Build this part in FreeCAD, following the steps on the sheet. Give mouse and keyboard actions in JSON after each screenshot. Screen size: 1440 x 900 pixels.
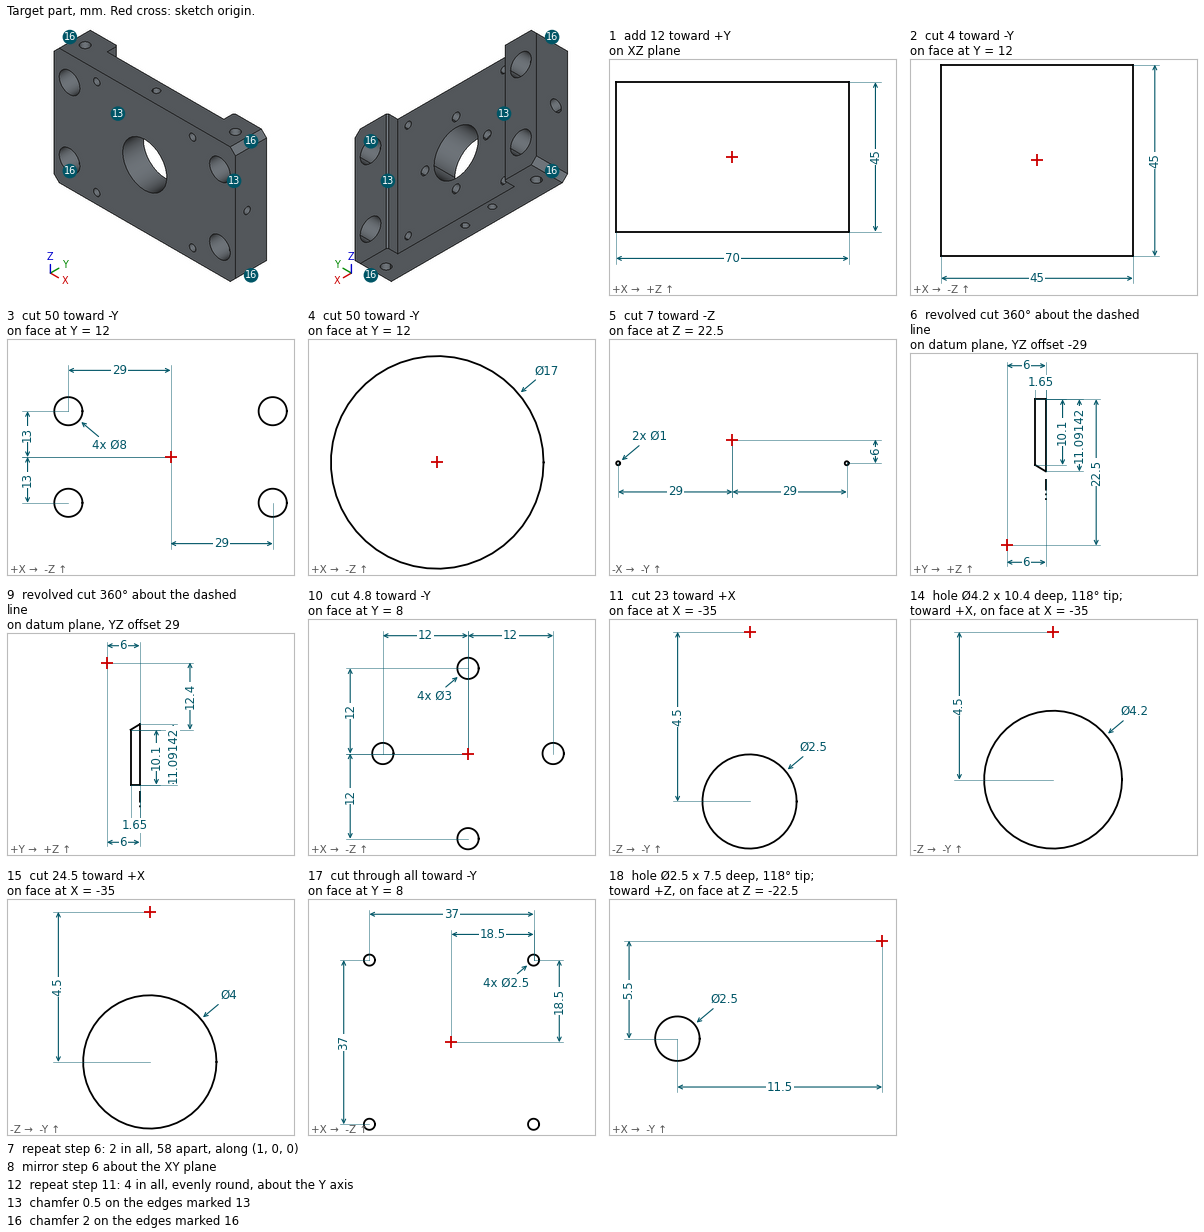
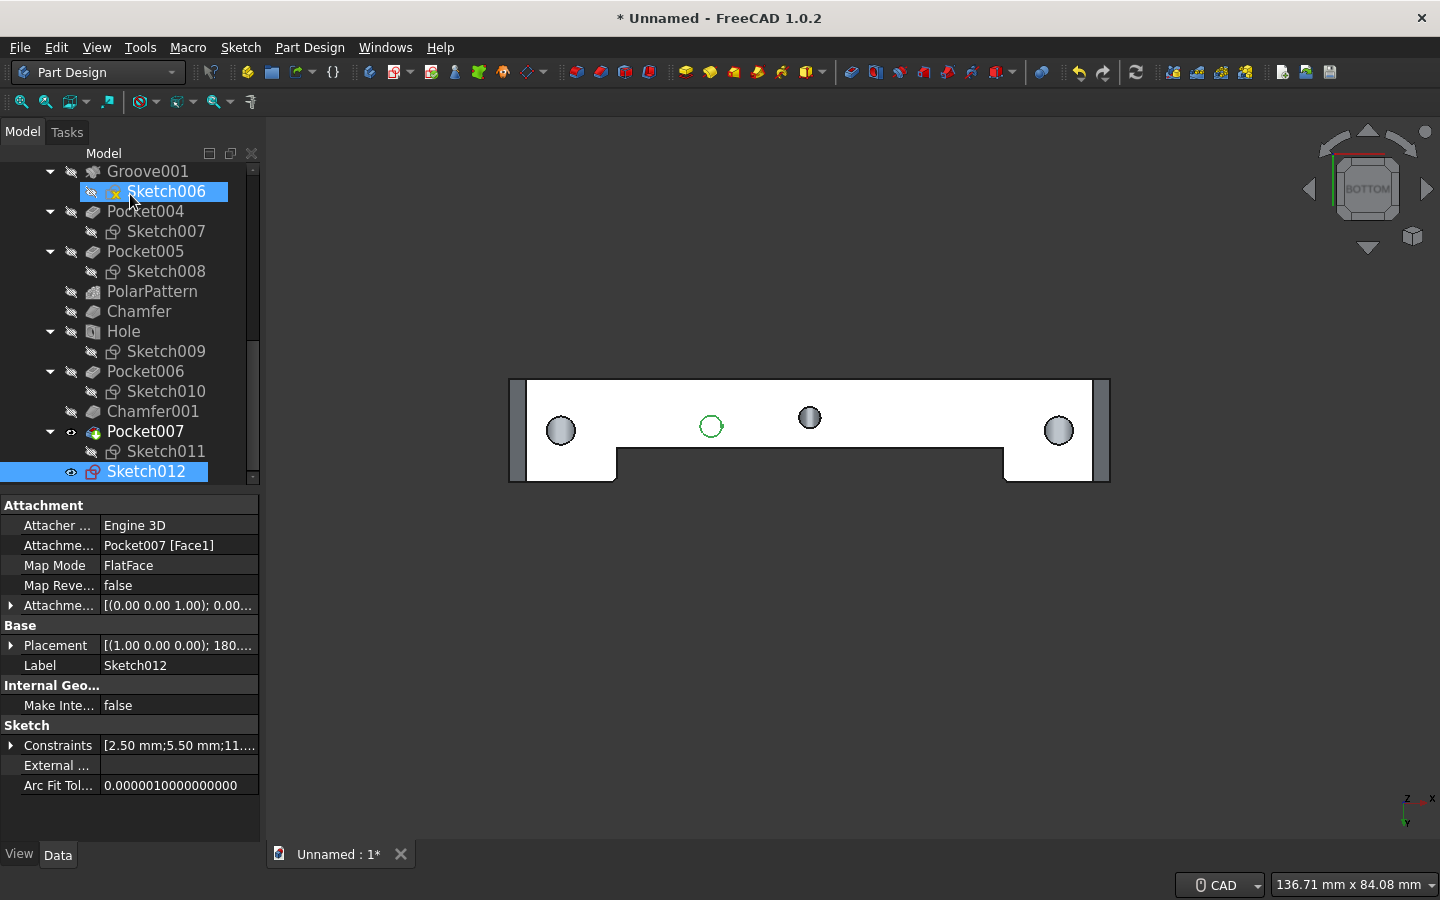
{"action": "left_click", "coordinate": [876, 72]}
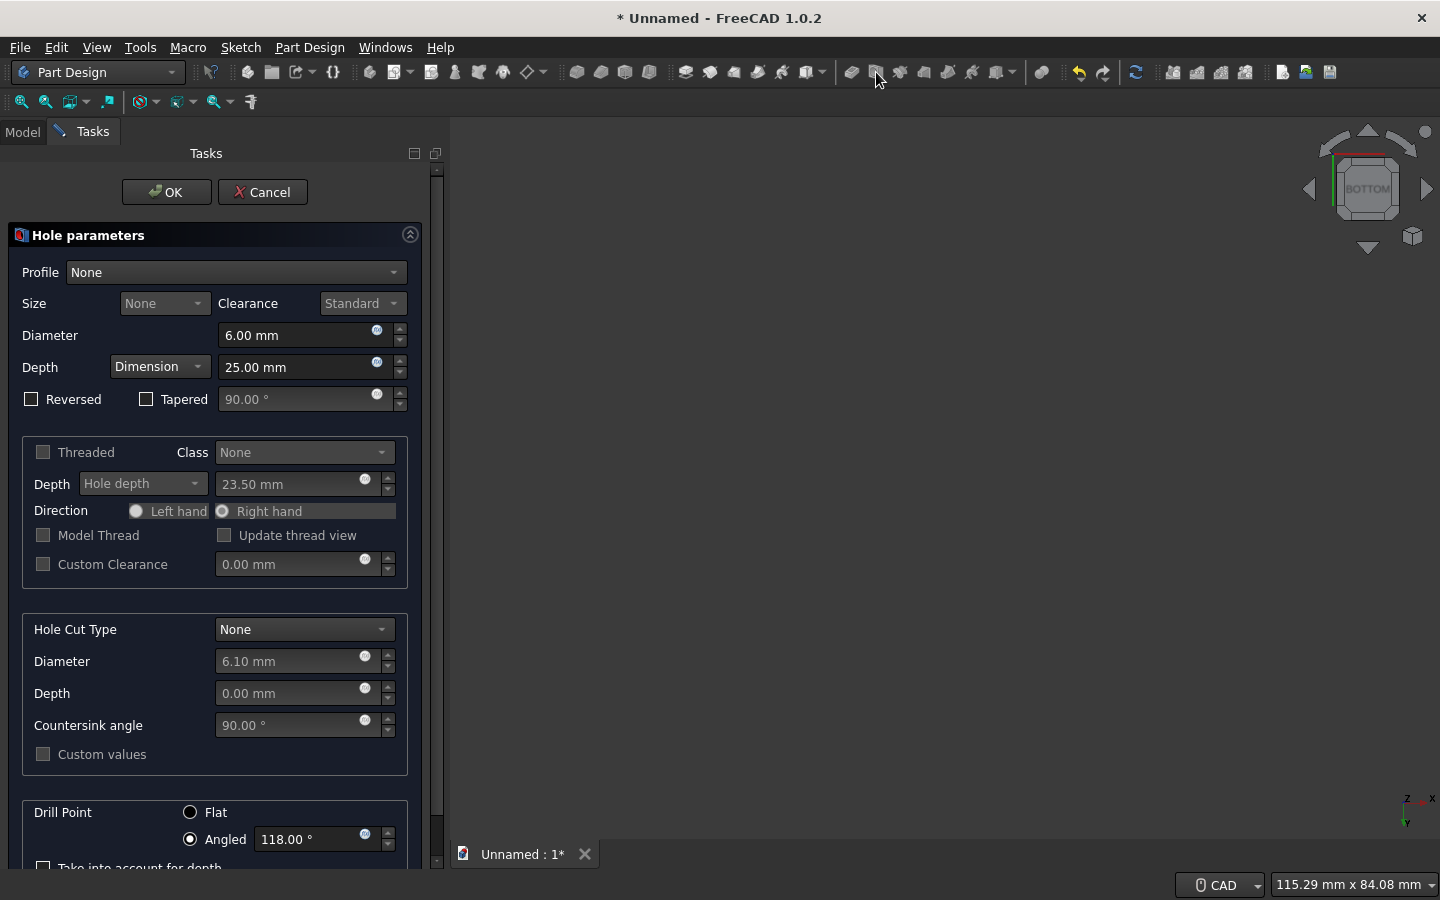
{"action": "triple_click", "coordinate": [305, 335]}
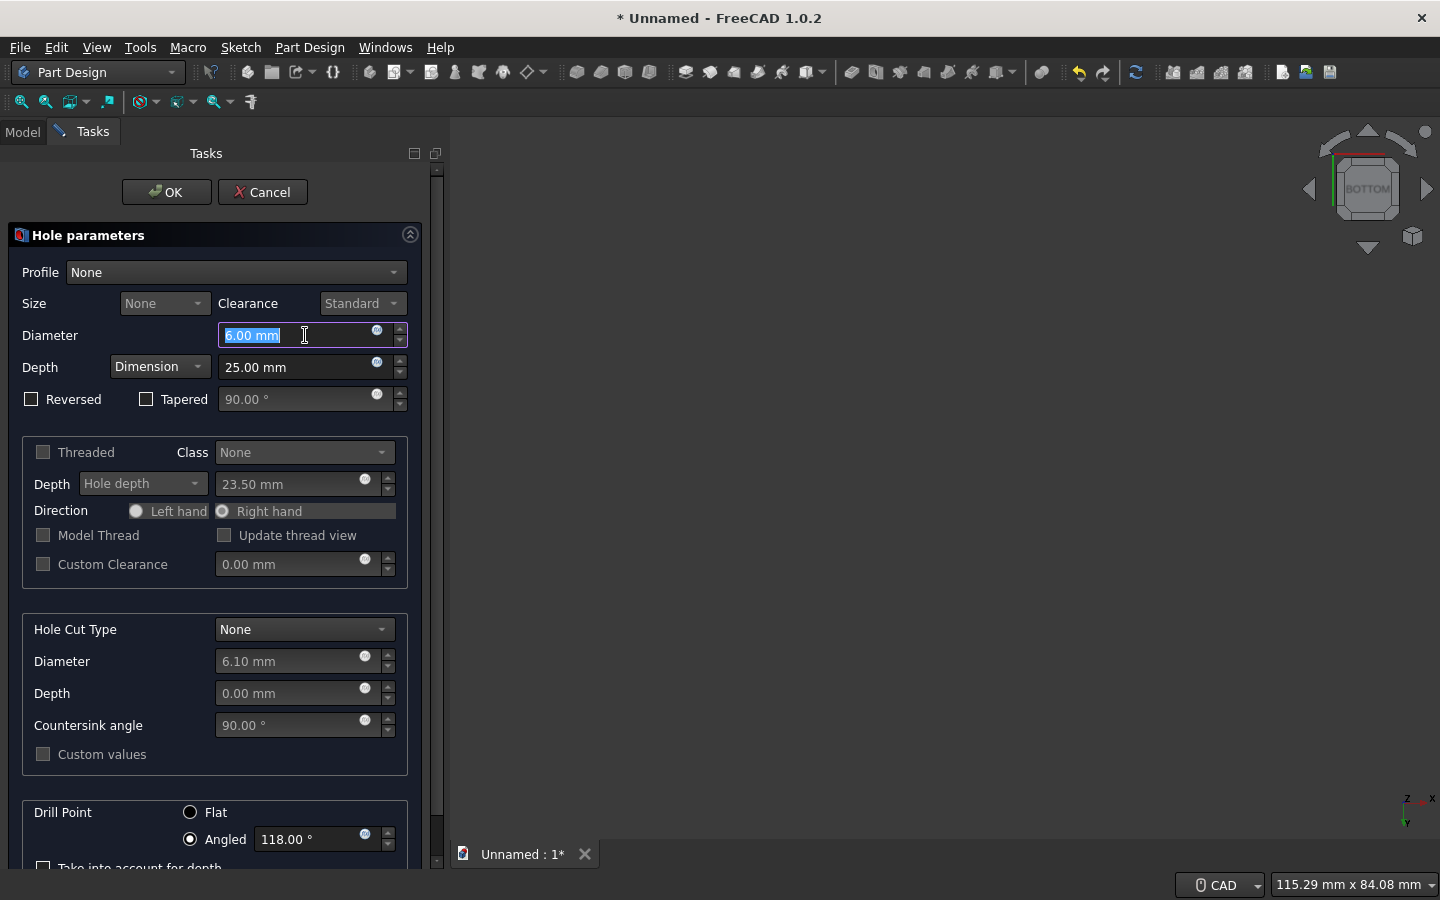
{"action": "type", "text": "2.5"}
{"action": "key", "text": "Tab"}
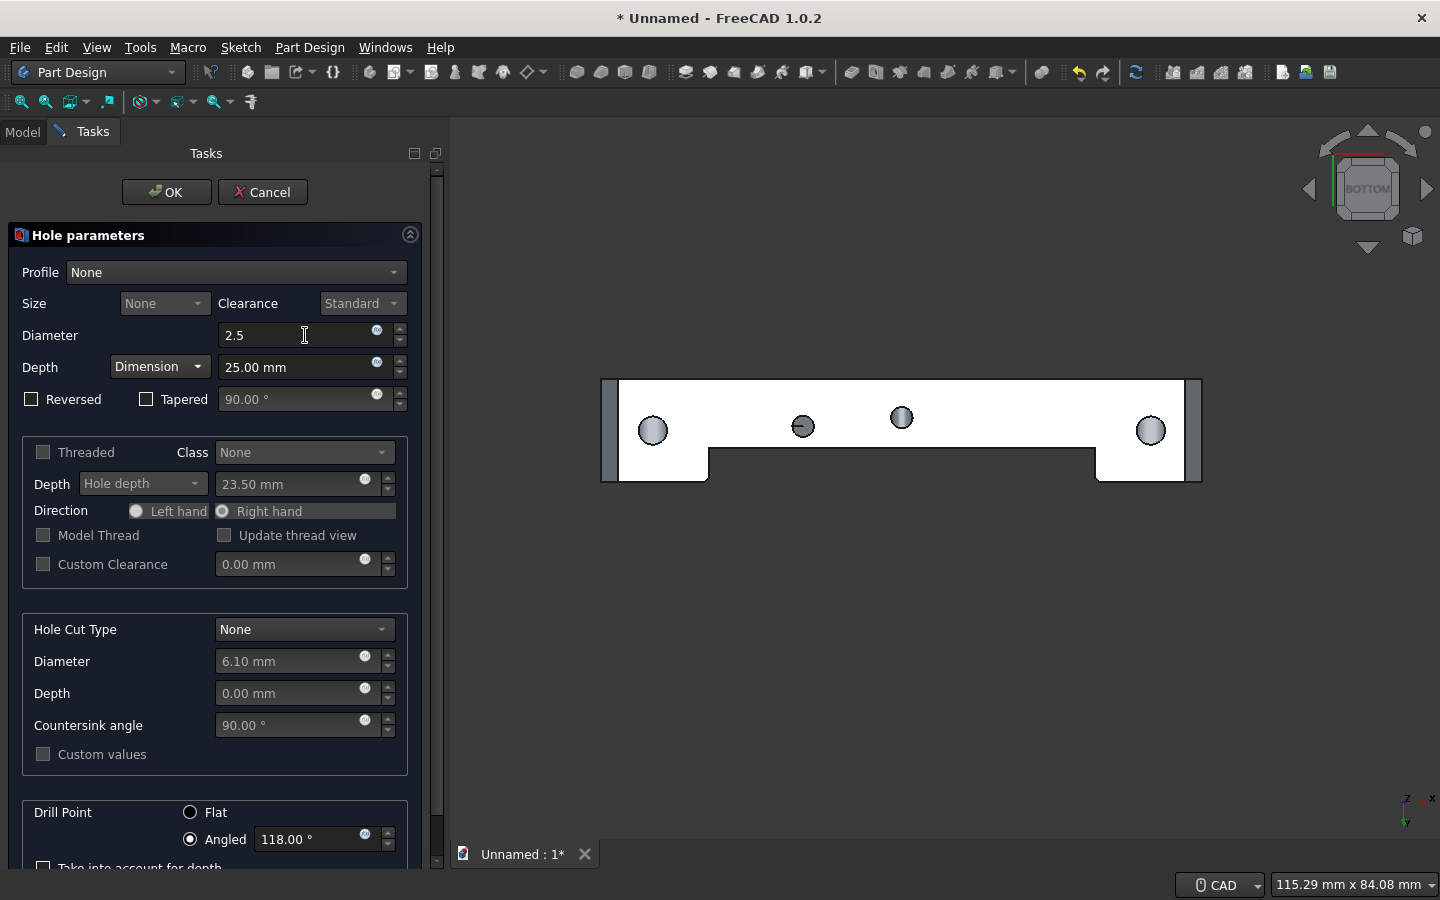
{"action": "triple_click", "coordinate": [305, 367]}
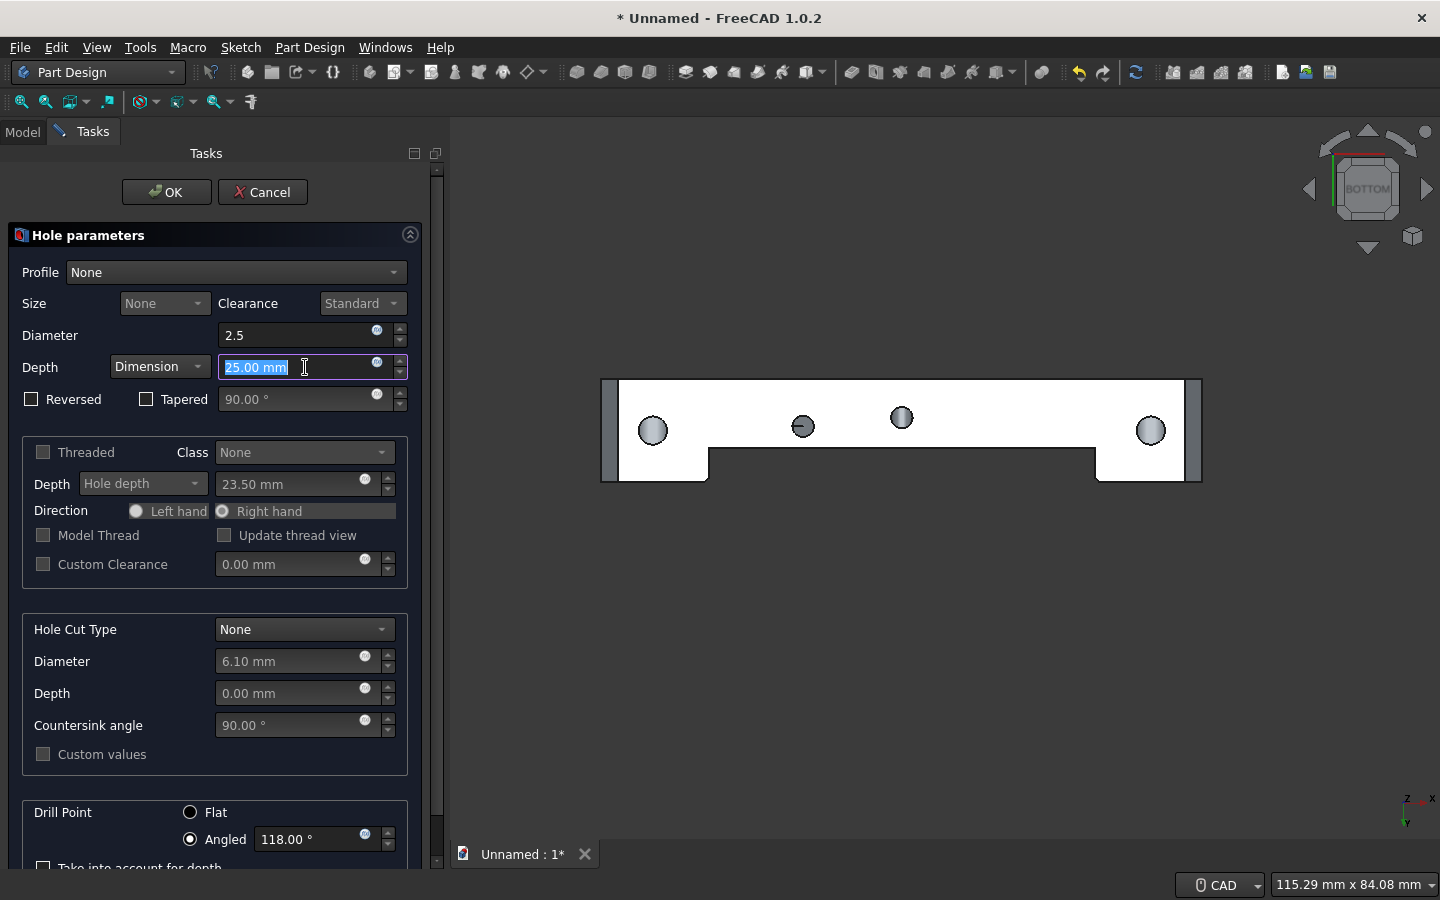
{"action": "type", "text": "7.5"}
{"action": "key", "text": "Tab"}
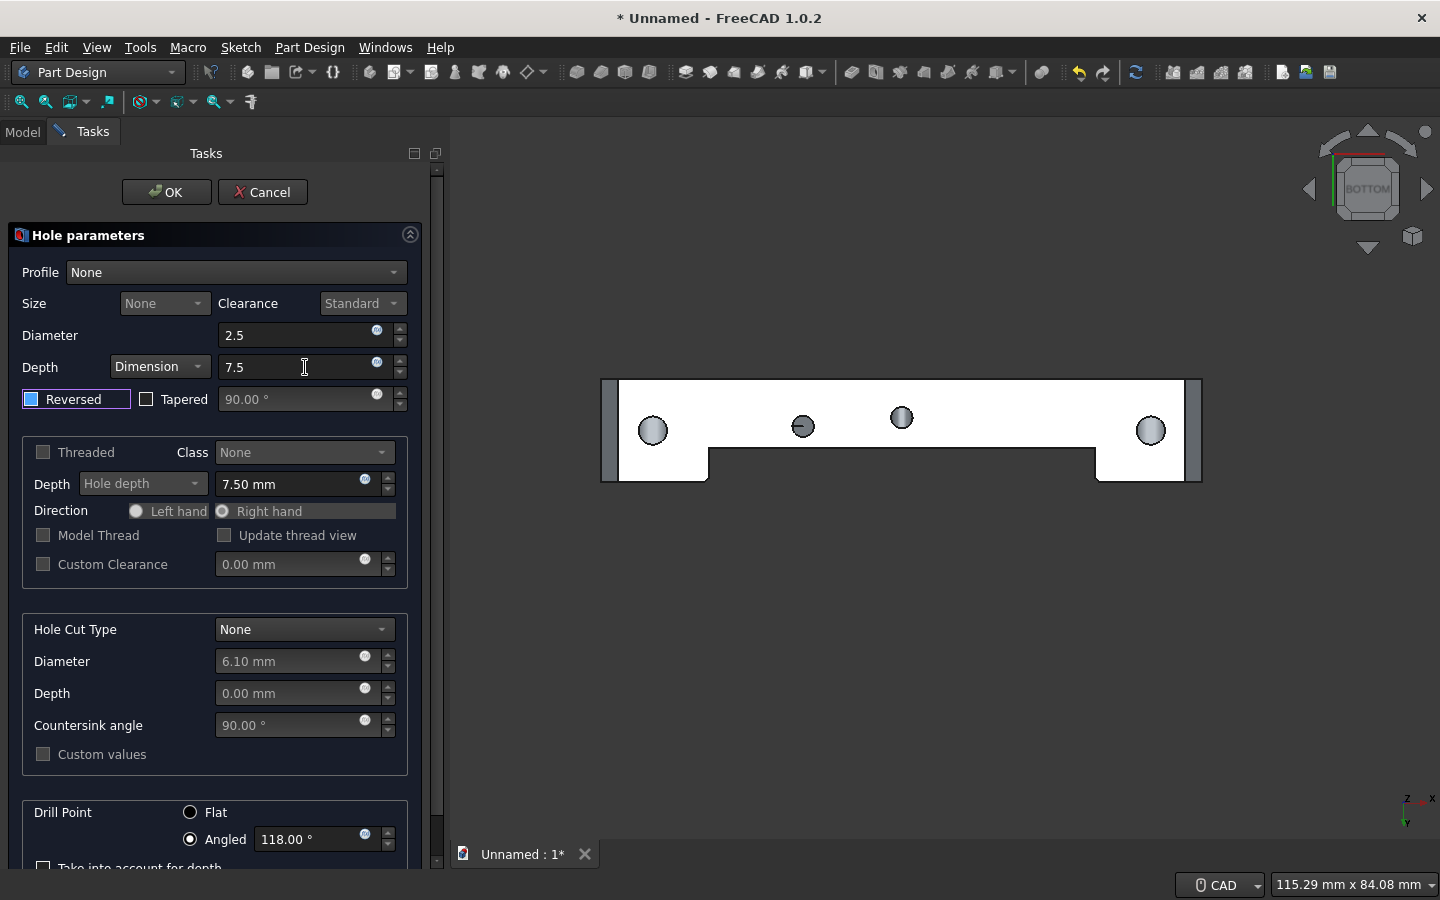
{"action": "left_click", "coordinate": [167, 192]}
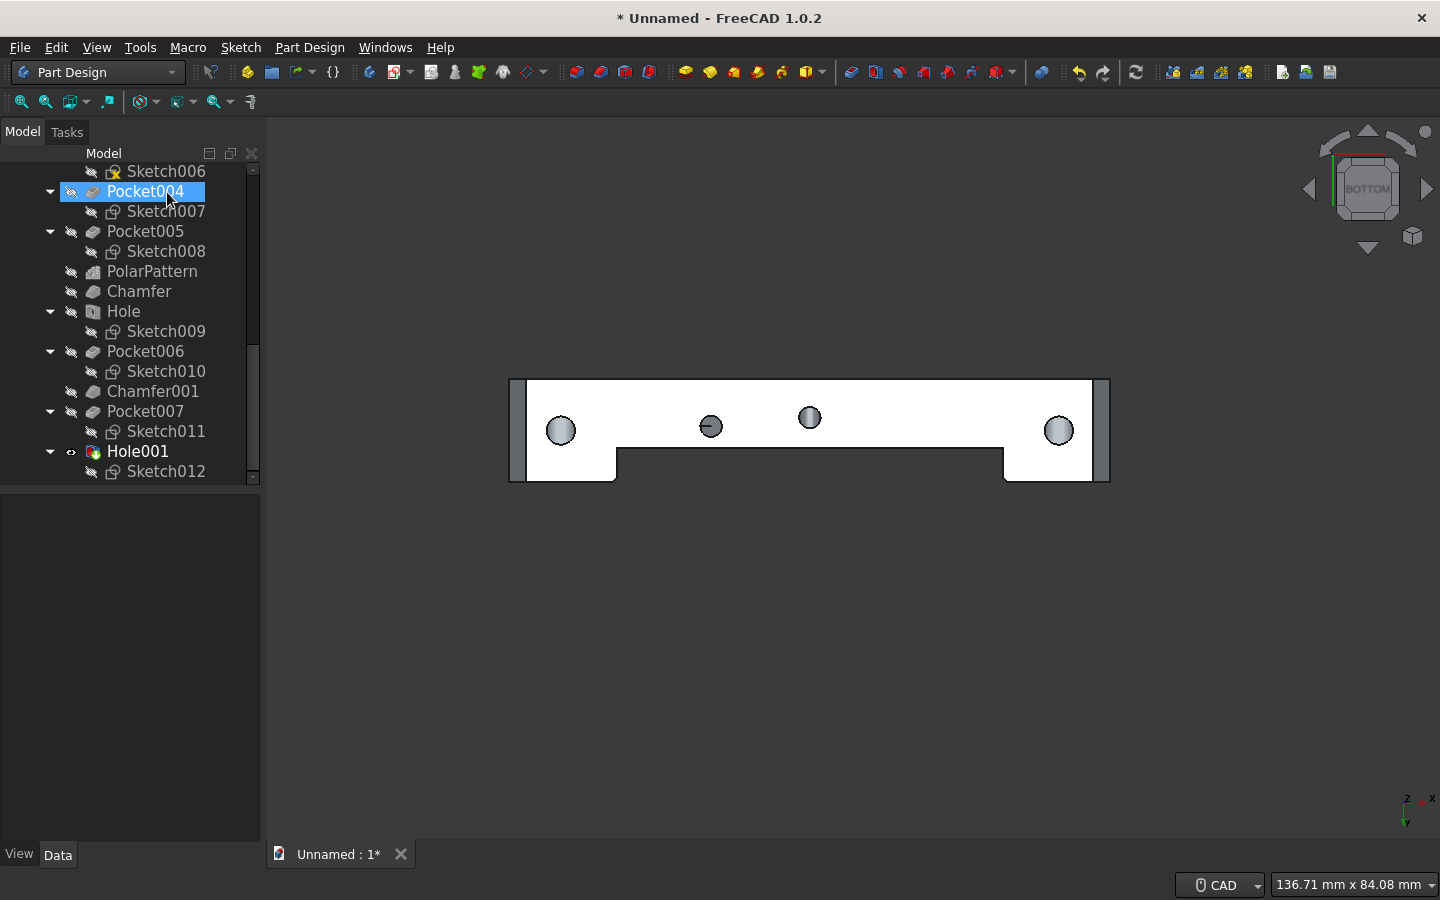
{"action": "key", "text": "0"}